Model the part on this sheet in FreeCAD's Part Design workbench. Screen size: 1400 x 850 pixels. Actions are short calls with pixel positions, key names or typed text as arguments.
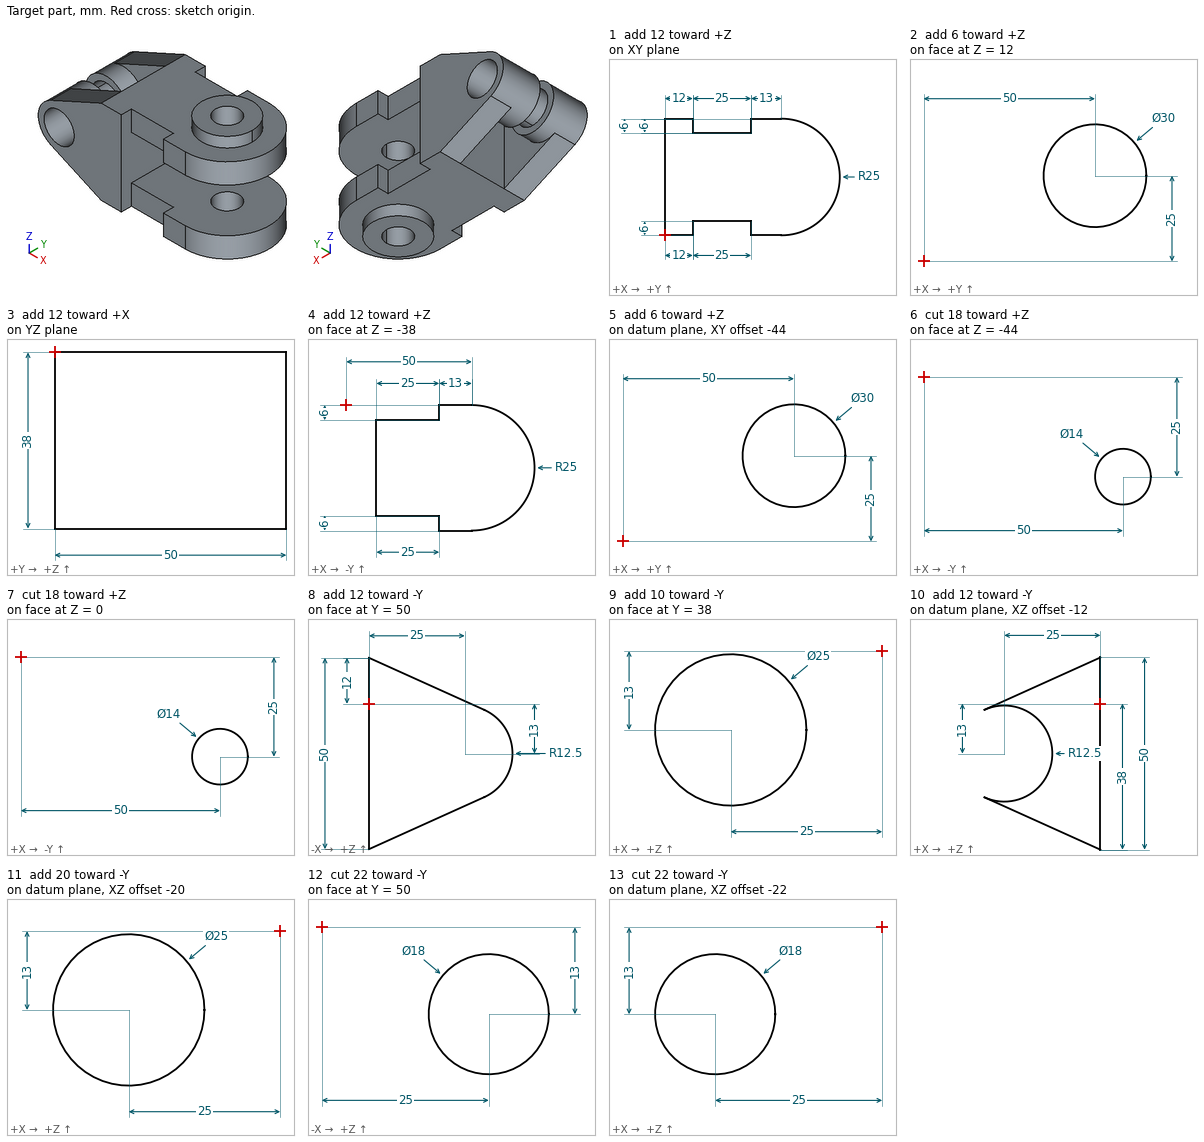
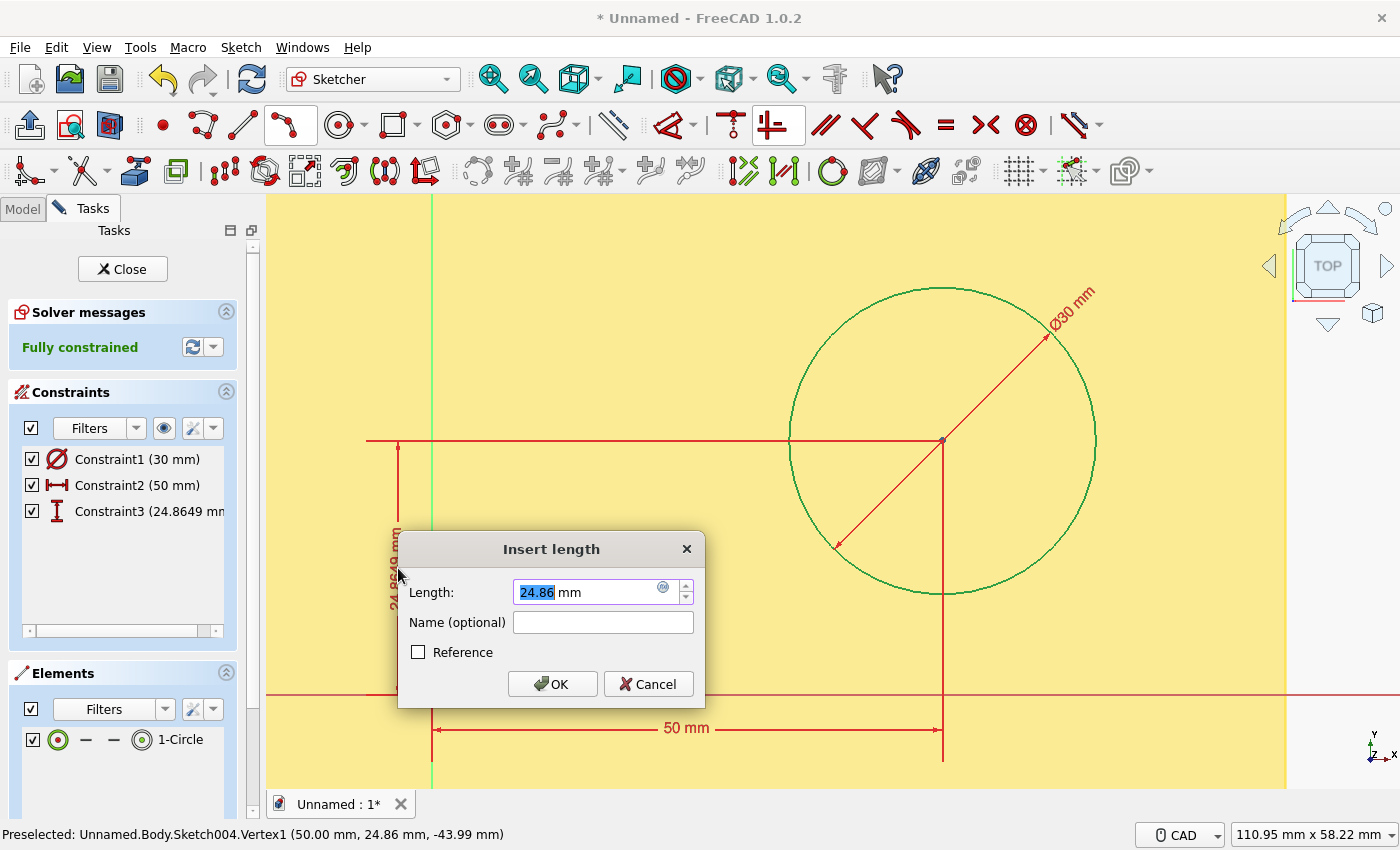
text(25)
key(Return)
key(Escape)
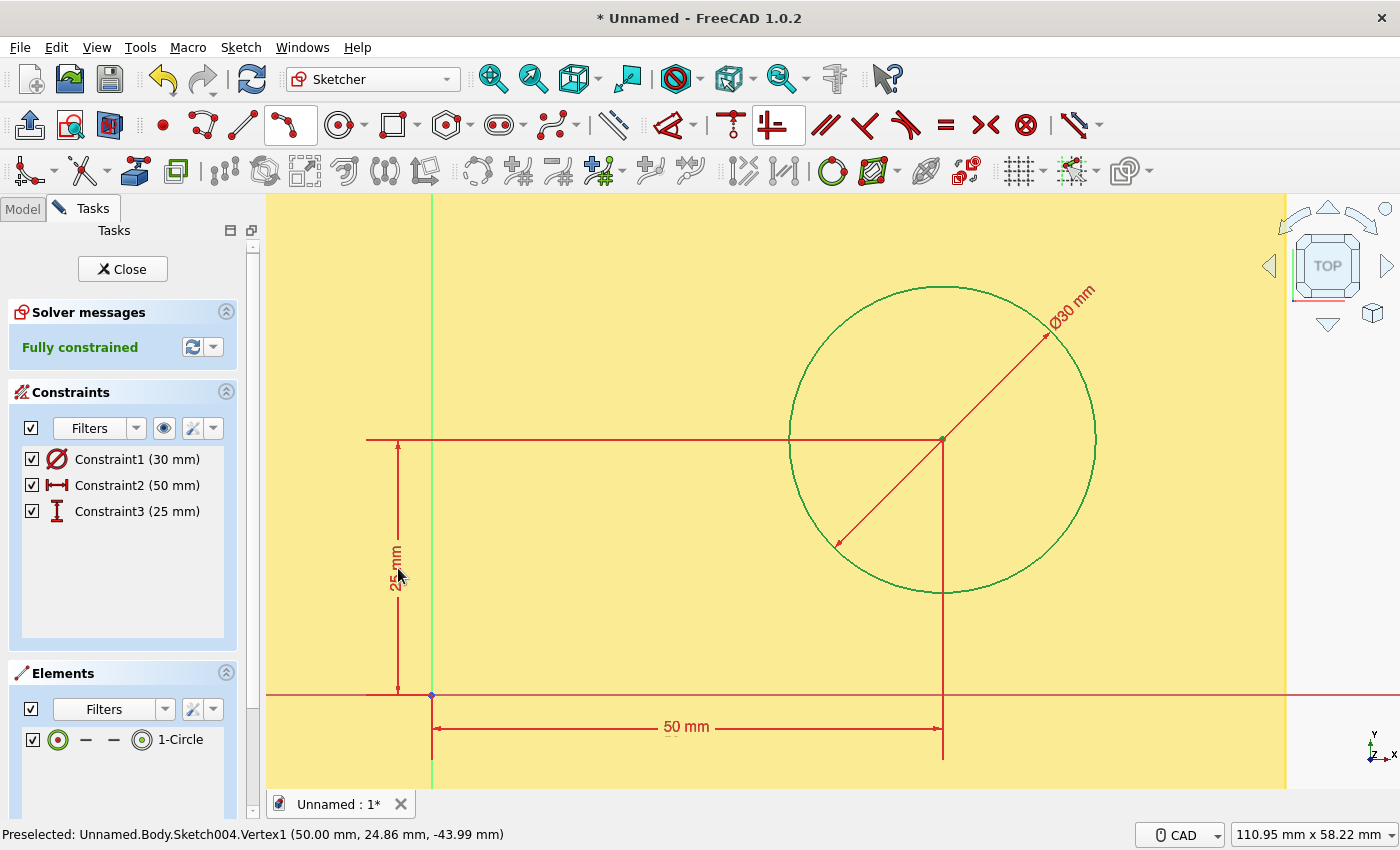
click(123, 269)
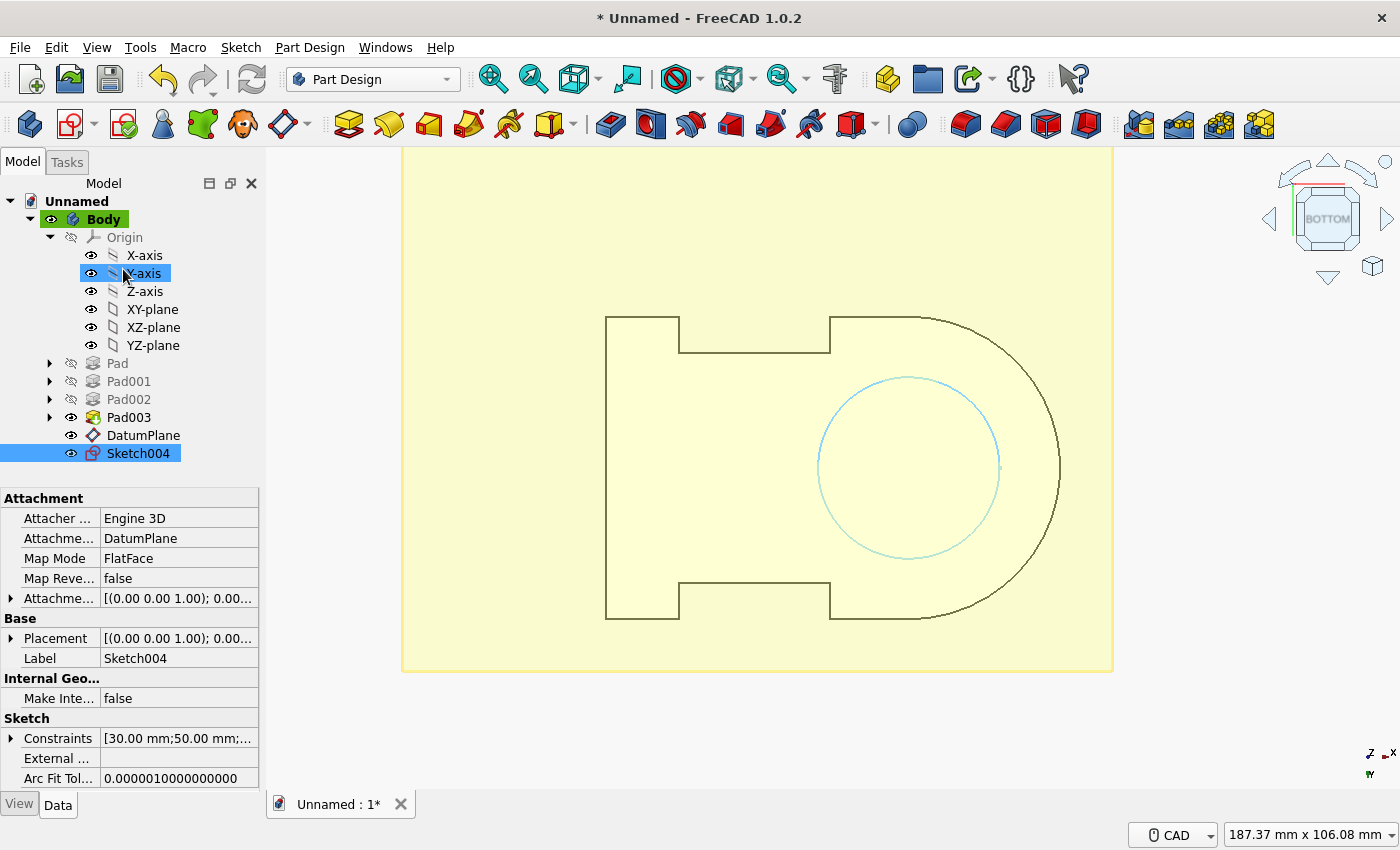
click(350, 124)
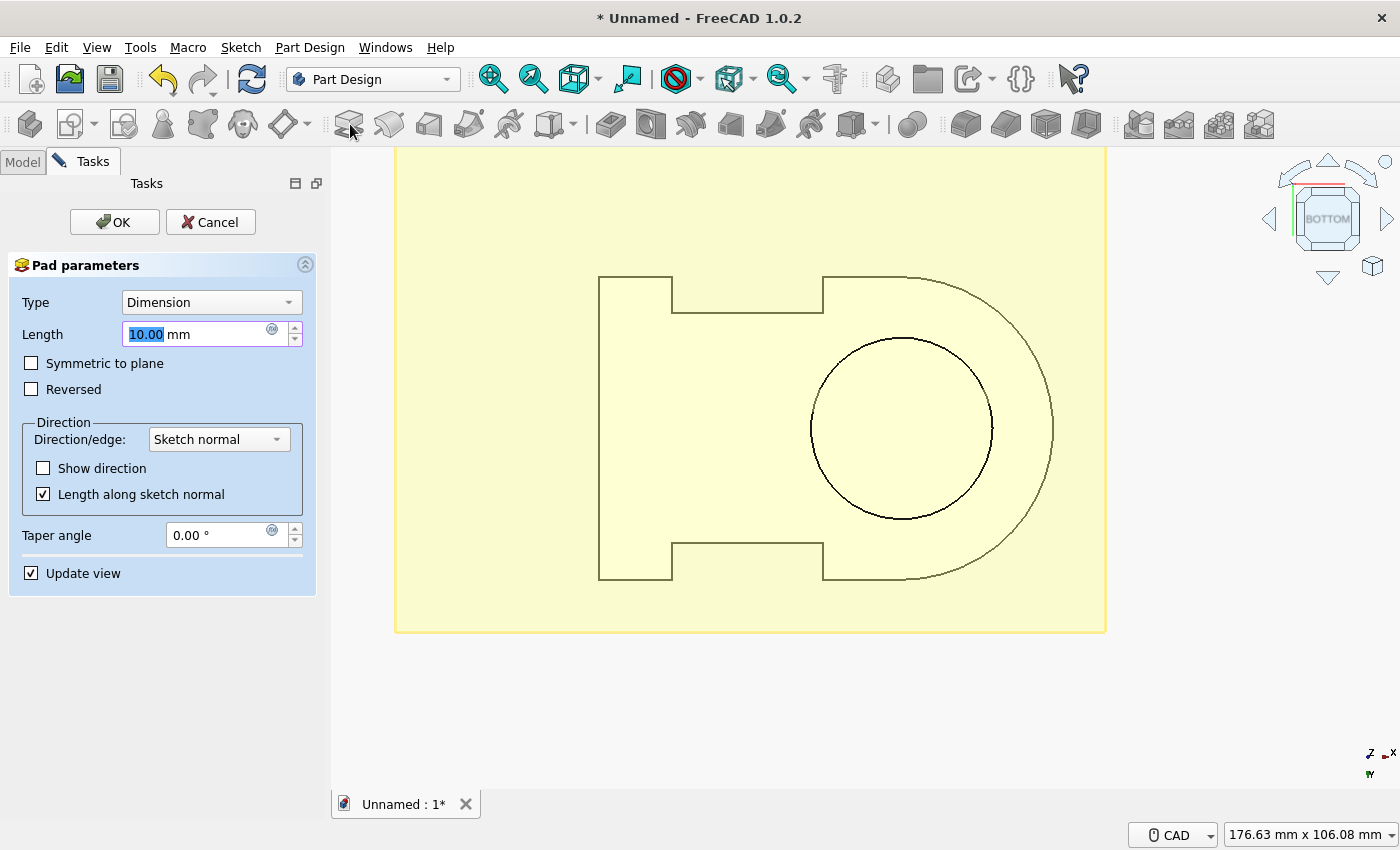
text(6)
key(Tab)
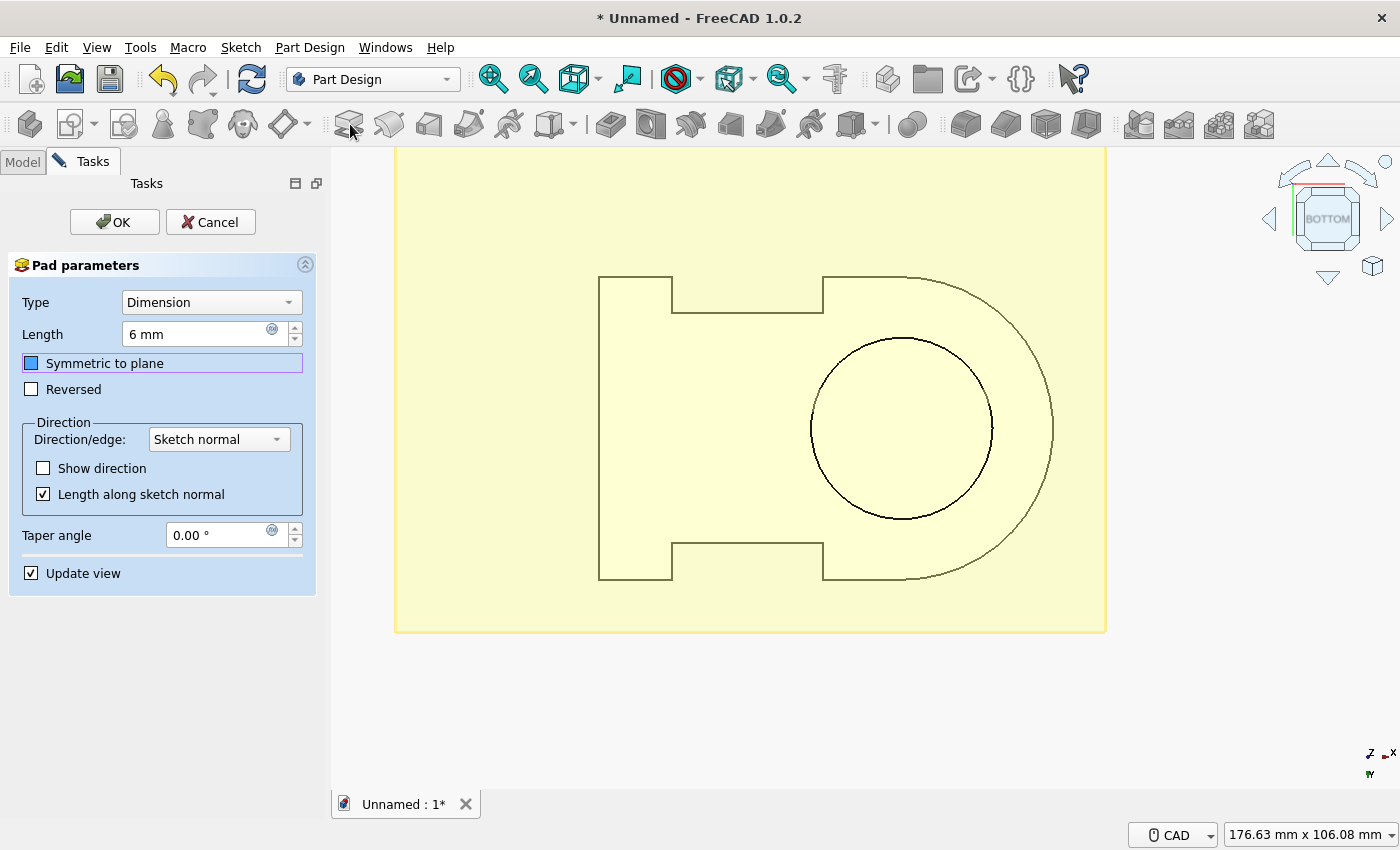
click(115, 222)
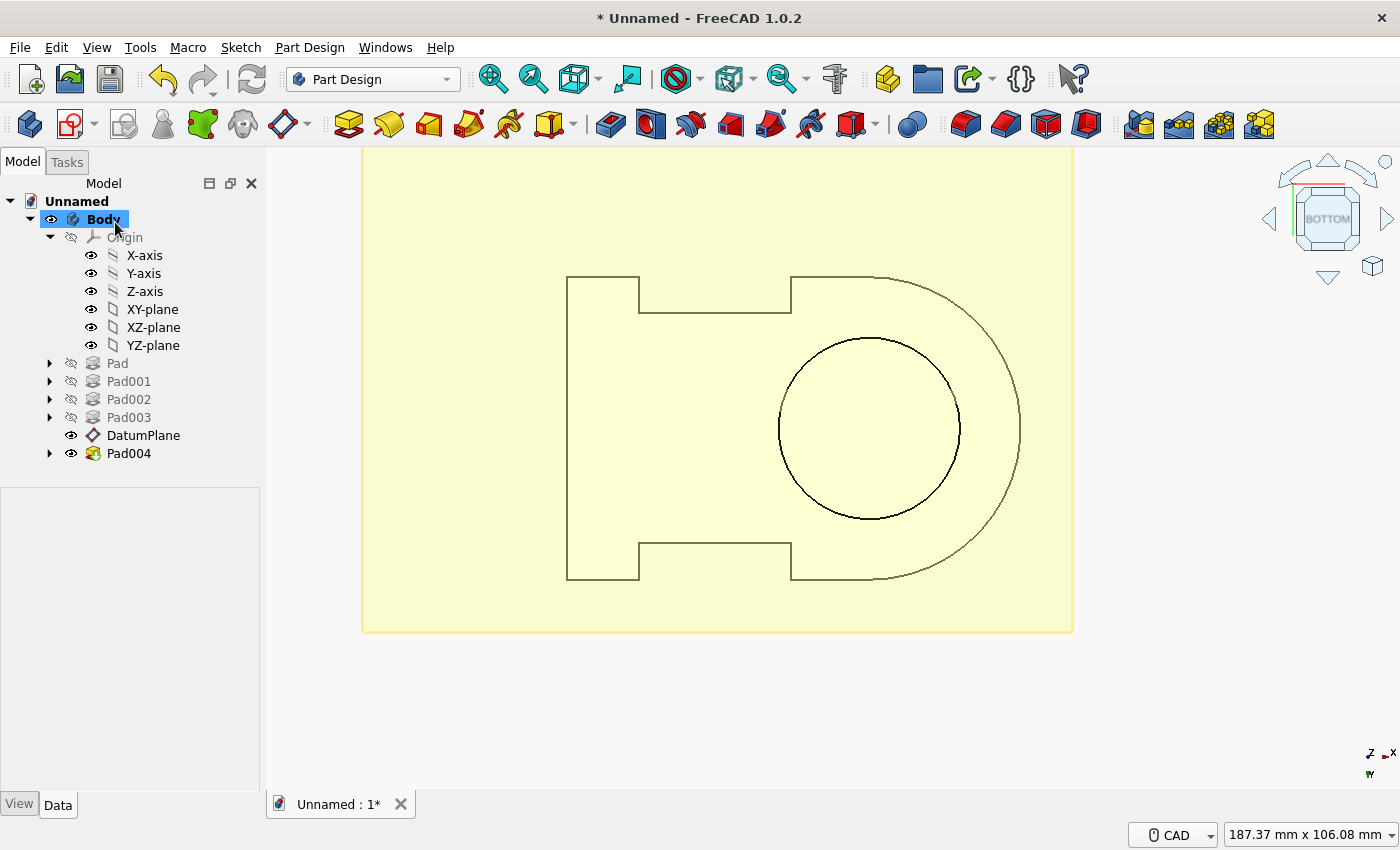
click(116, 435)
key(space)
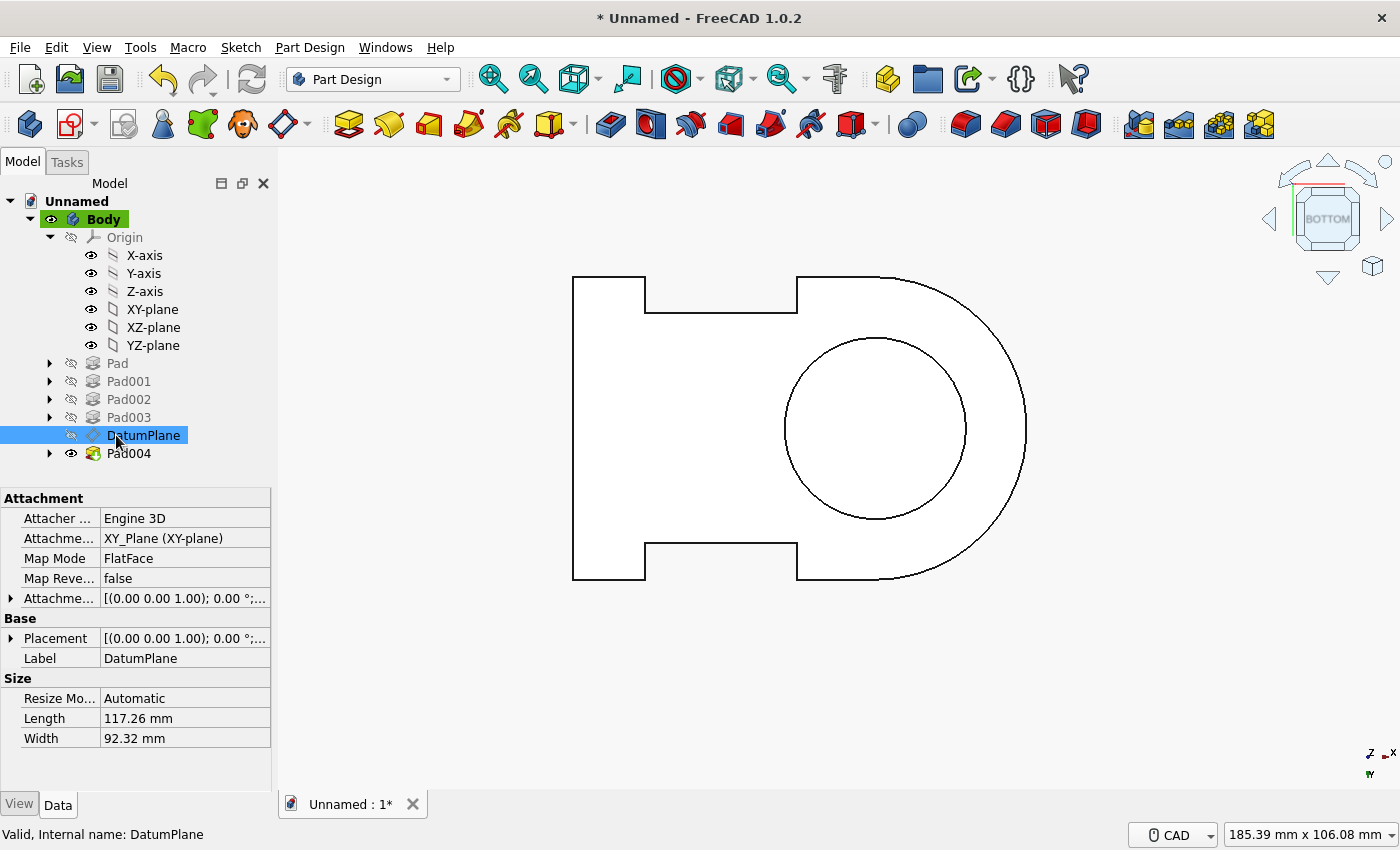
click(875, 427)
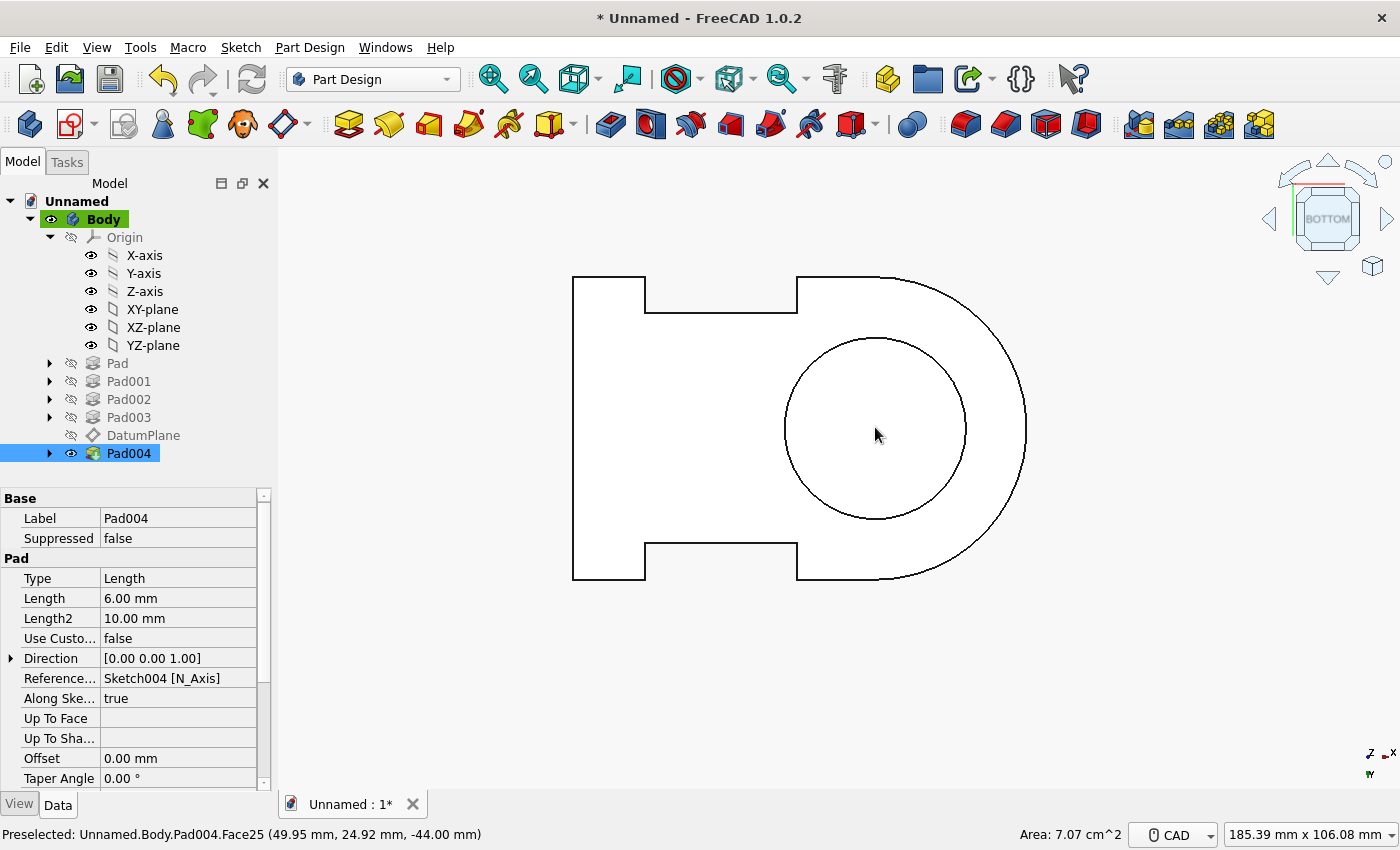
click(70, 124)